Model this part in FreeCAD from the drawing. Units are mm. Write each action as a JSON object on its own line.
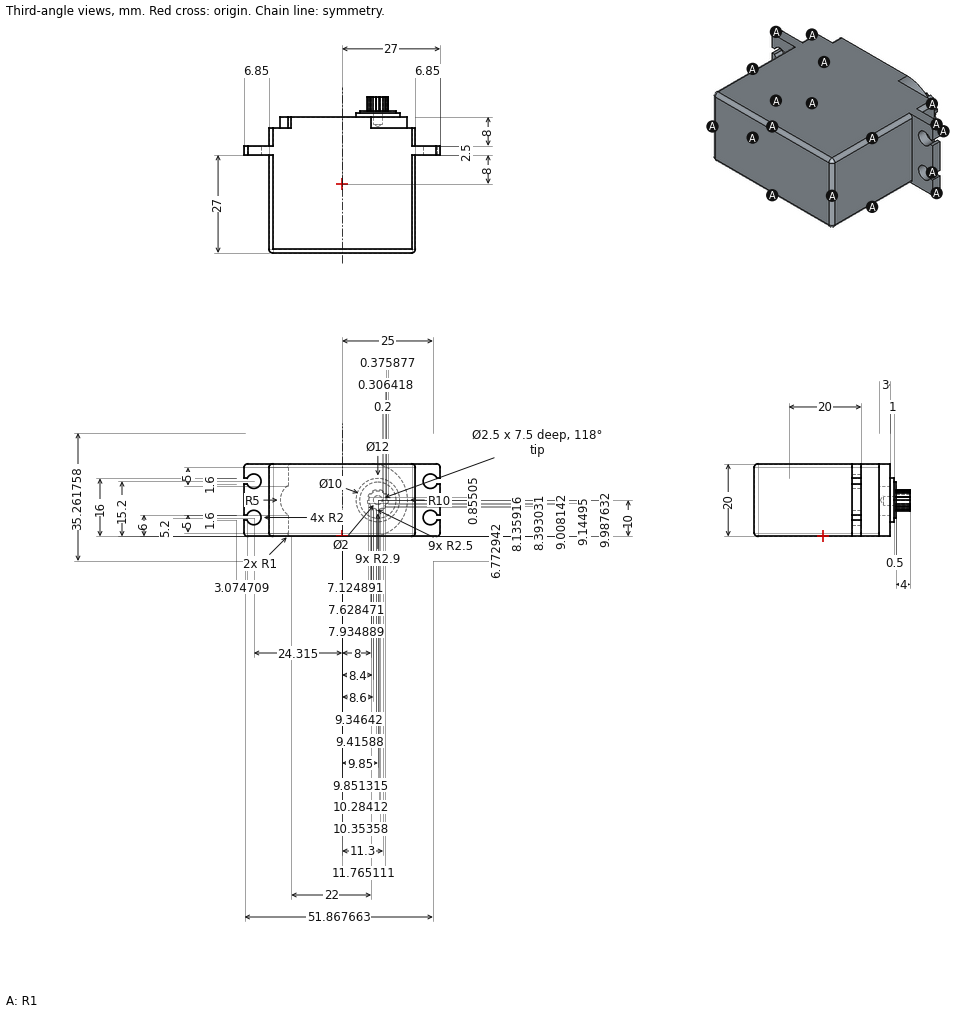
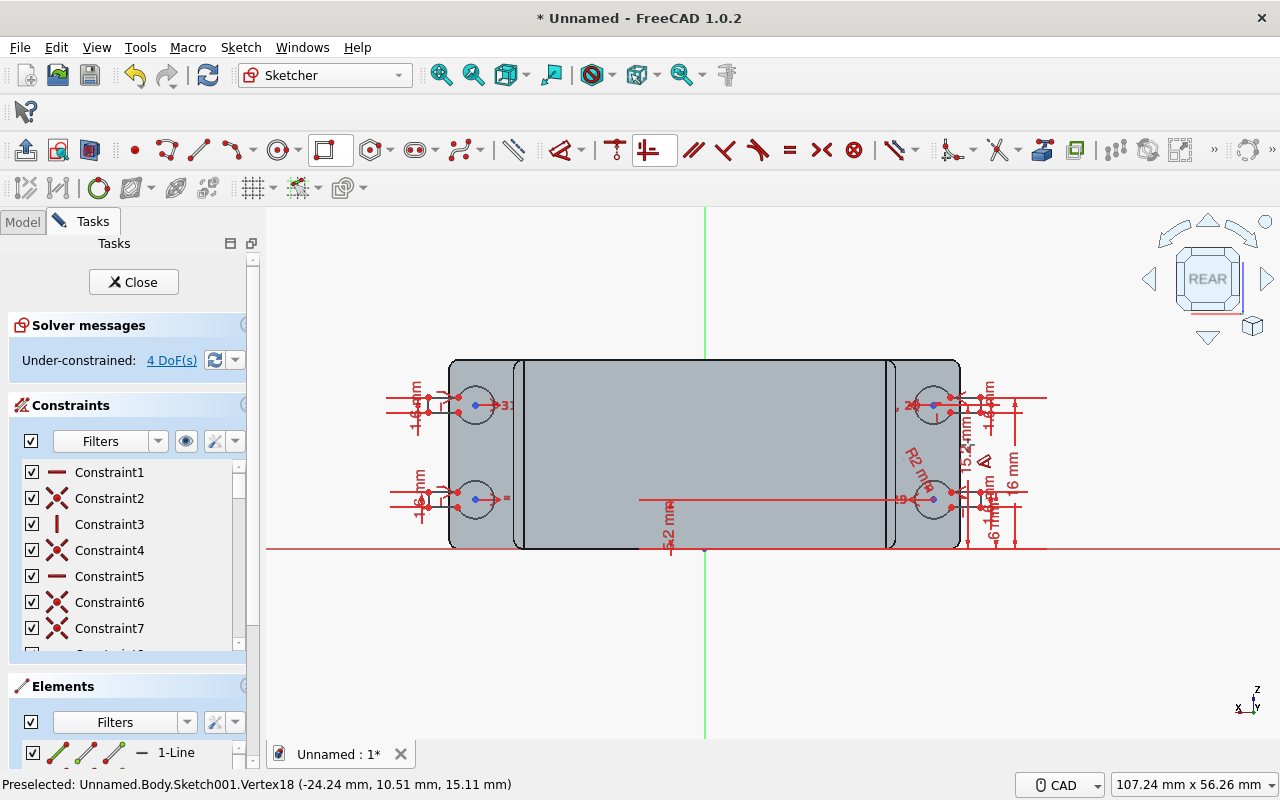
{"action": "left_click", "coordinate": [934, 500]}
{"action": "left_click", "coordinate": [819, 583]}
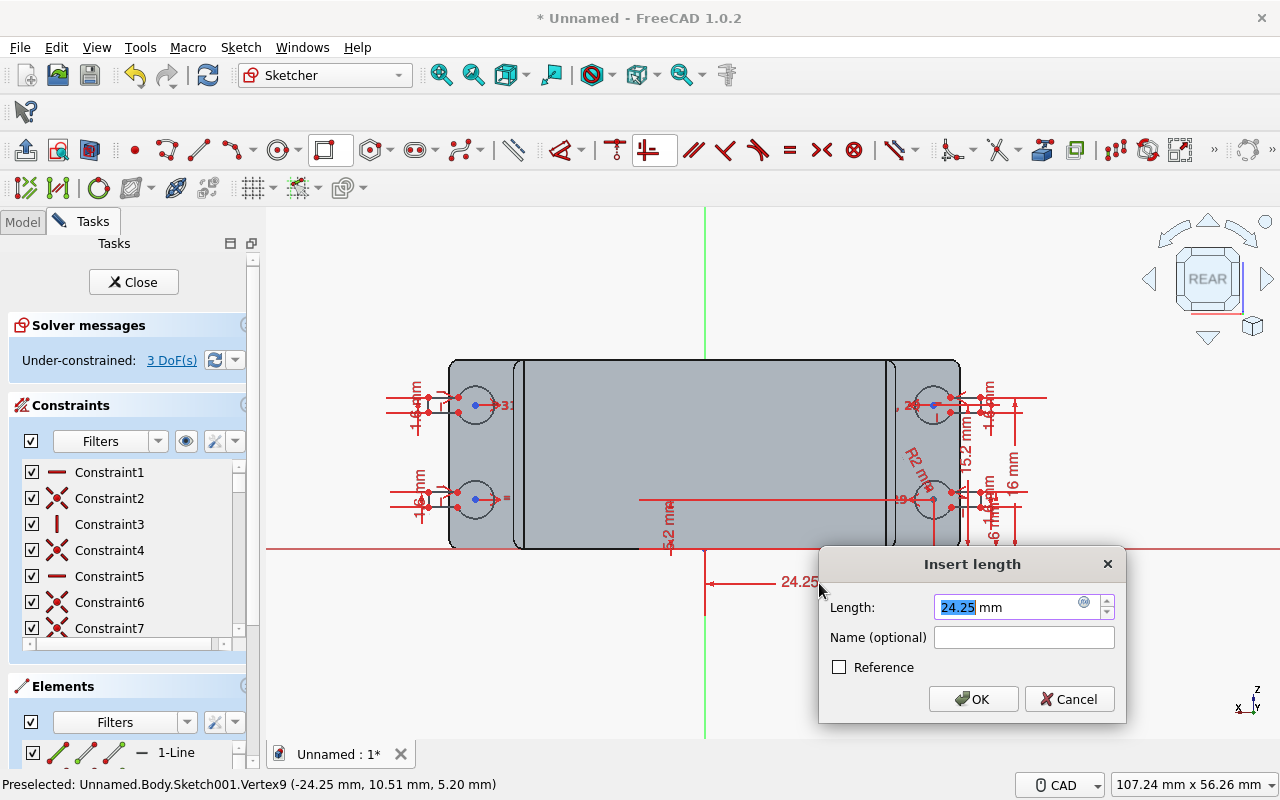
{"action": "type", "text": "24.315"}
{"action": "key", "text": "Return"}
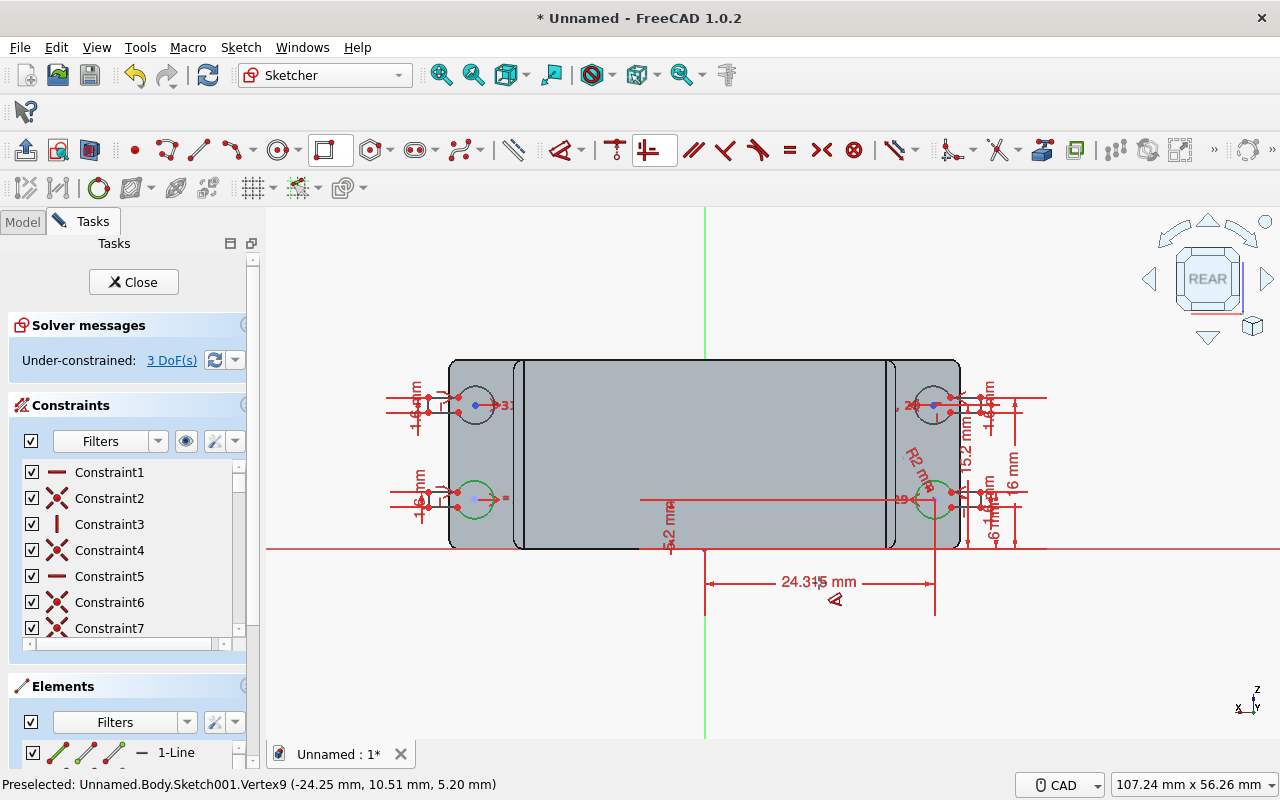
{"action": "left_click", "coordinate": [934, 405]}
{"action": "left_click", "coordinate": [739, 583]}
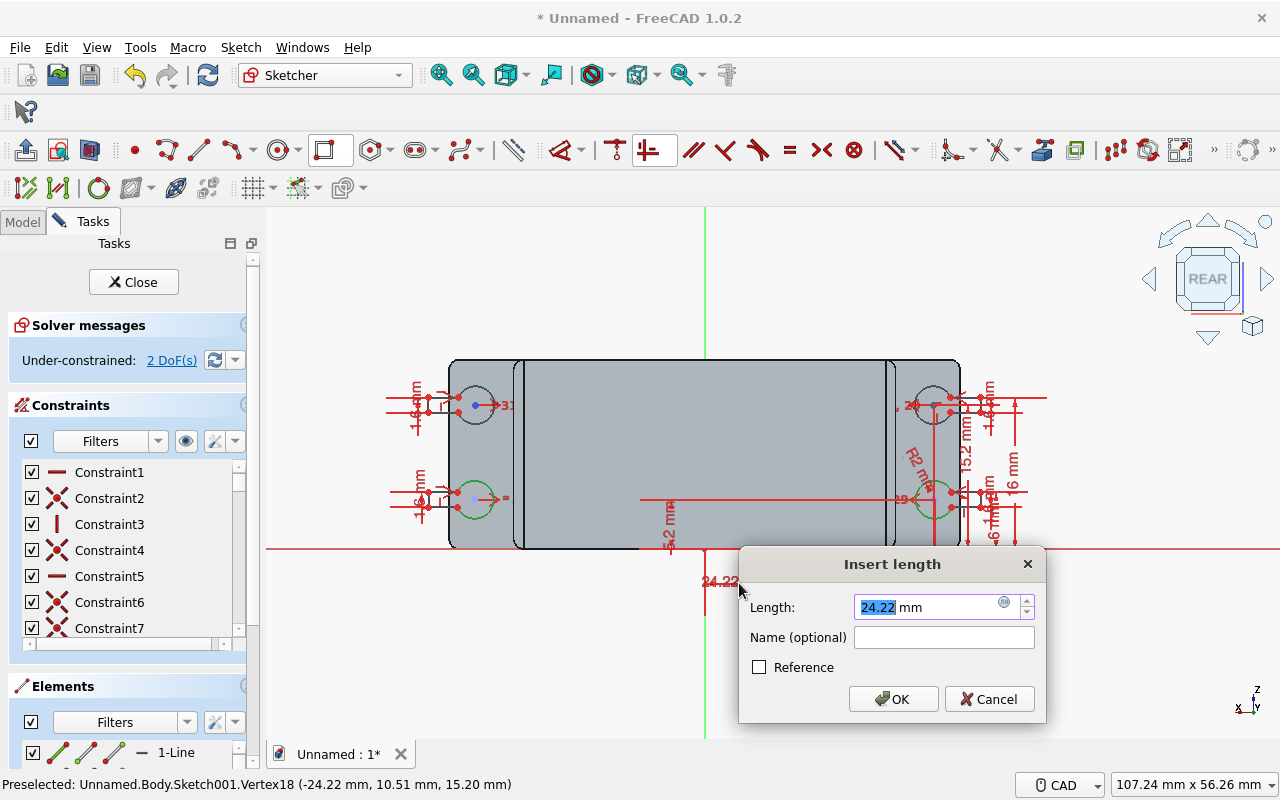
{"action": "type", "text": "24.315"}
{"action": "key", "text": "Return"}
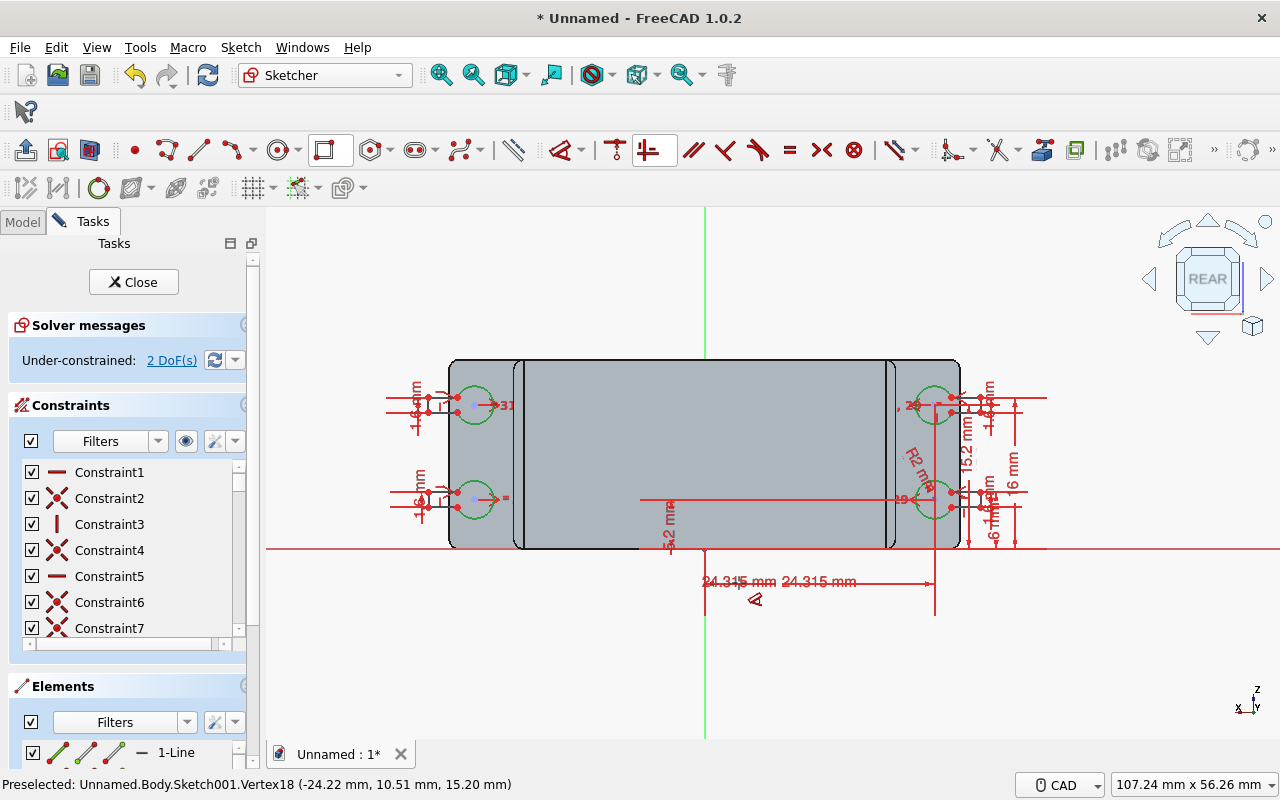
{"action": "scroll", "coordinate": [963, 507], "scroll_direction": "up", "scroll_amount": 2}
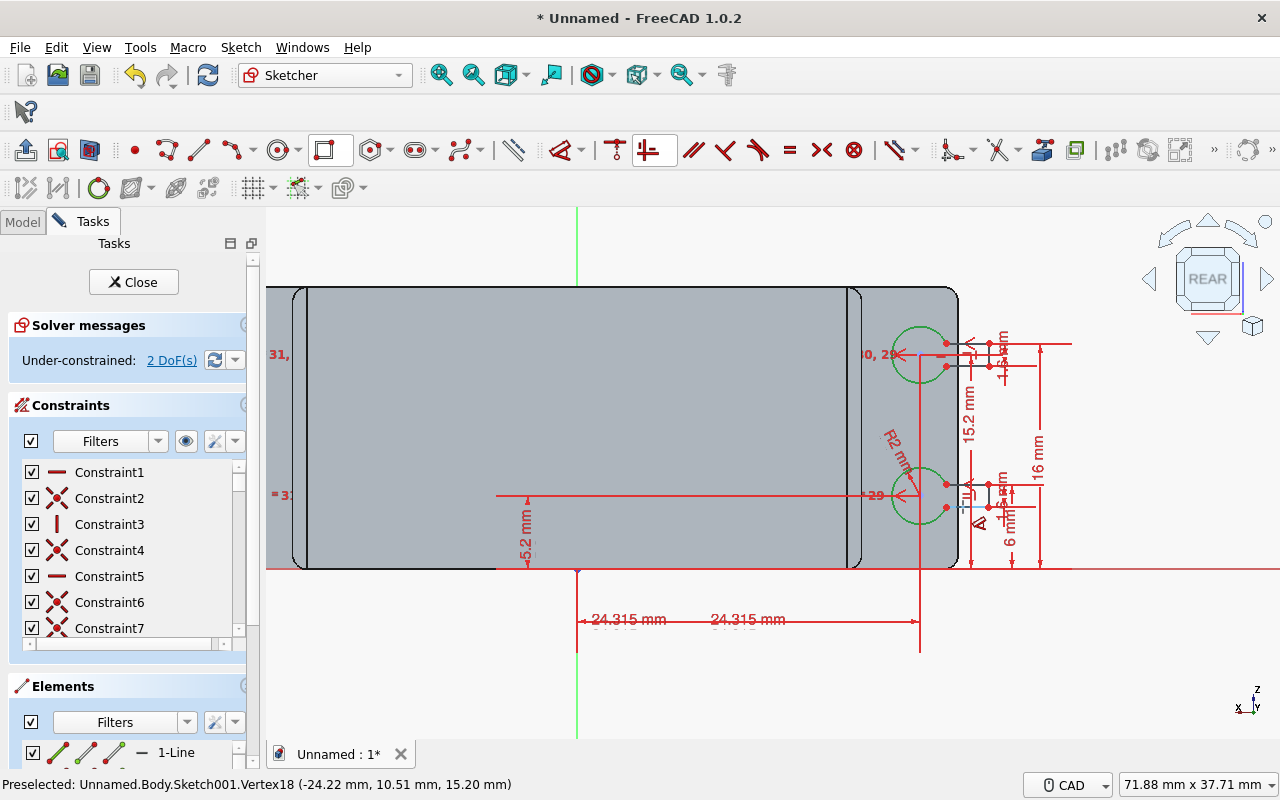
{"action": "left_click", "coordinate": [963, 507]}
{"action": "left_click", "coordinate": [968, 449]}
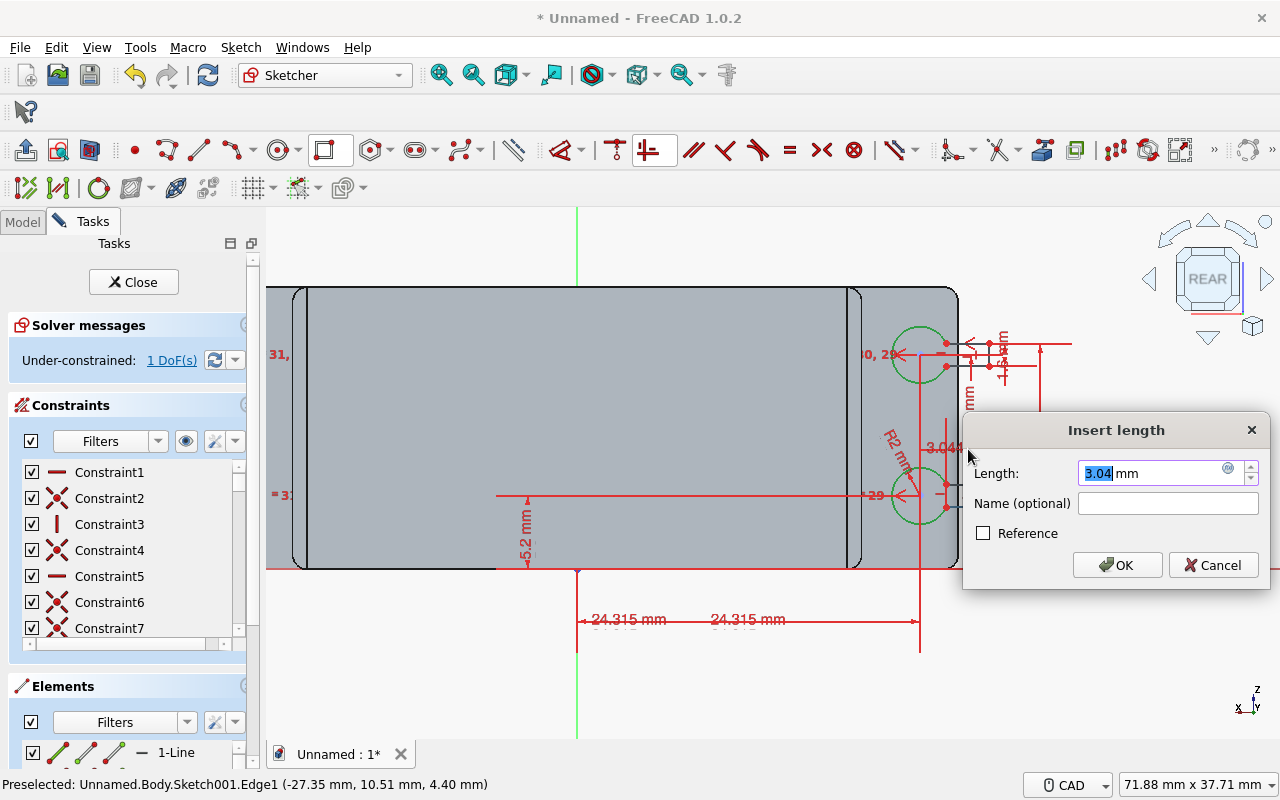
{"action": "type", "text": "3.074709"}
{"action": "key", "text": "Return"}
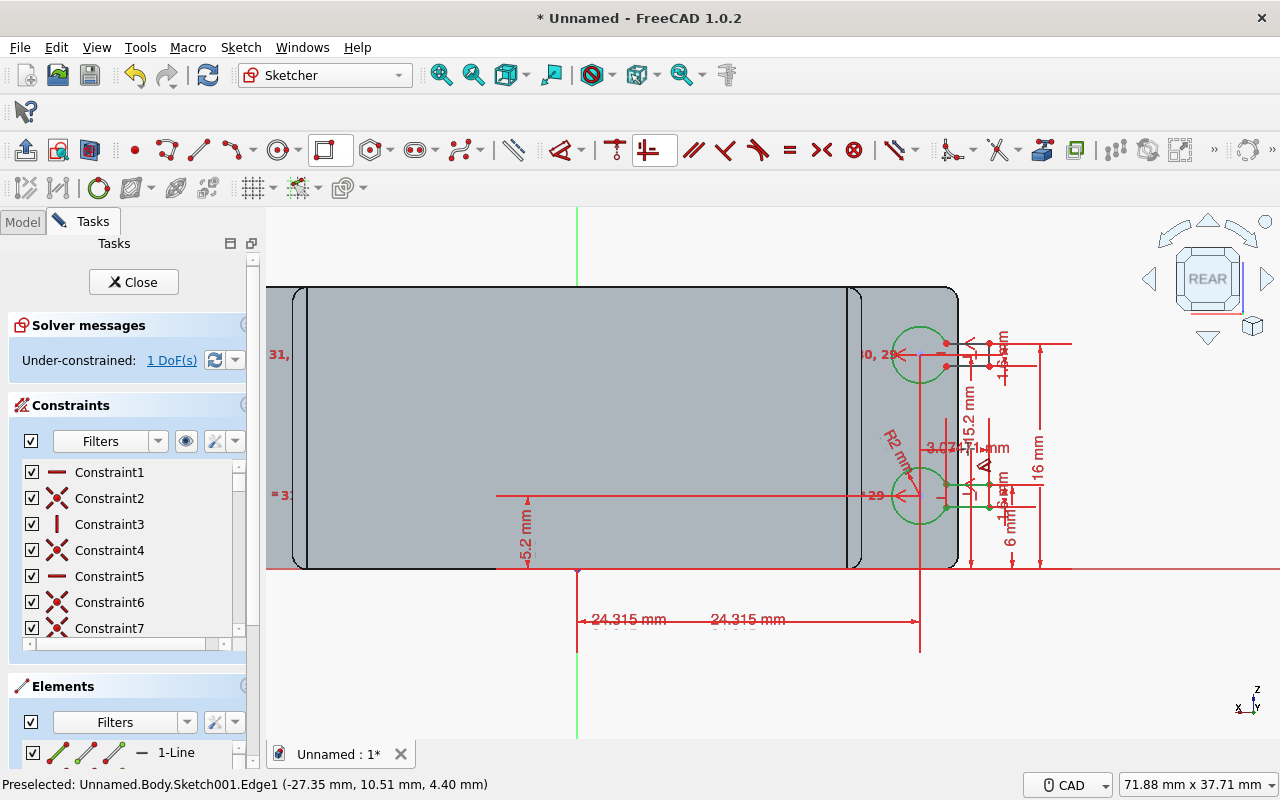
{"action": "left_click", "coordinate": [959, 366]}
{"action": "left_click", "coordinate": [968, 308]}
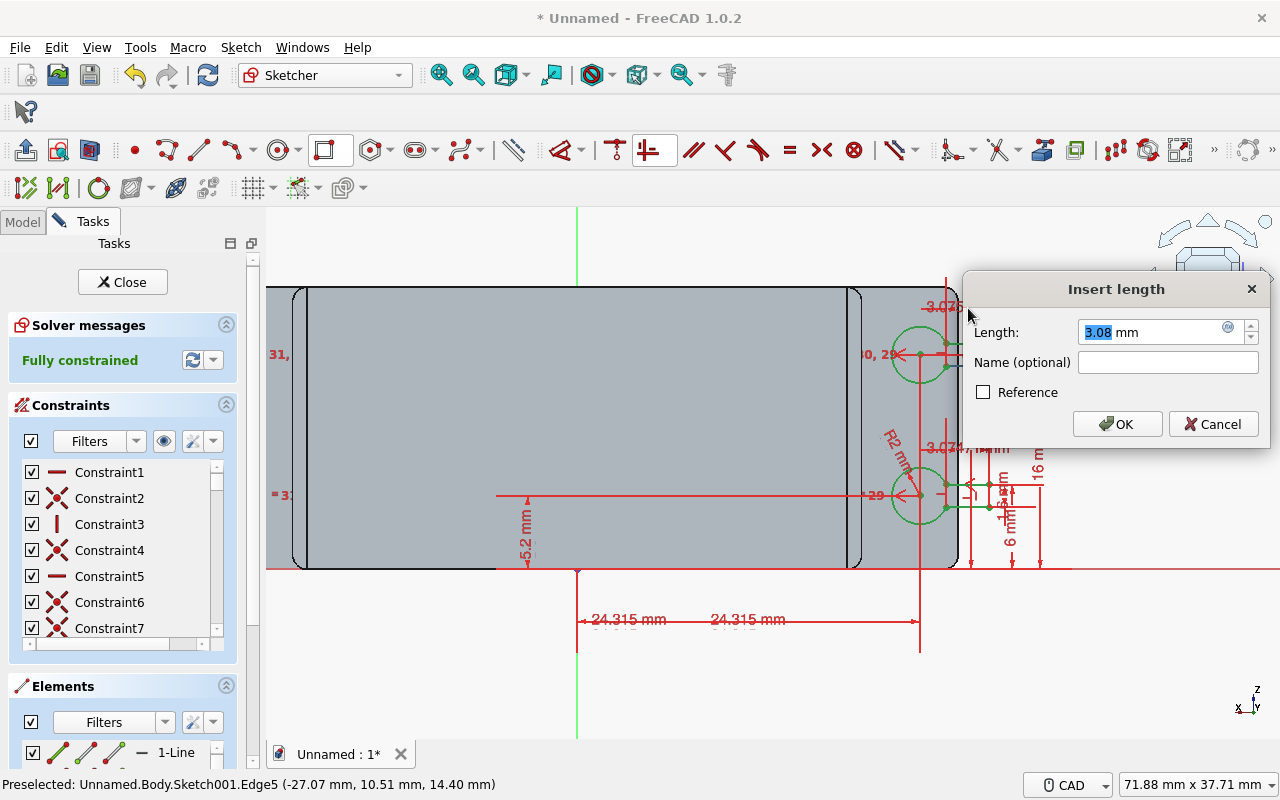
{"action": "type", "text": "3.074709"}
{"action": "key", "text": "Return"}
{"action": "key", "text": "Escape"}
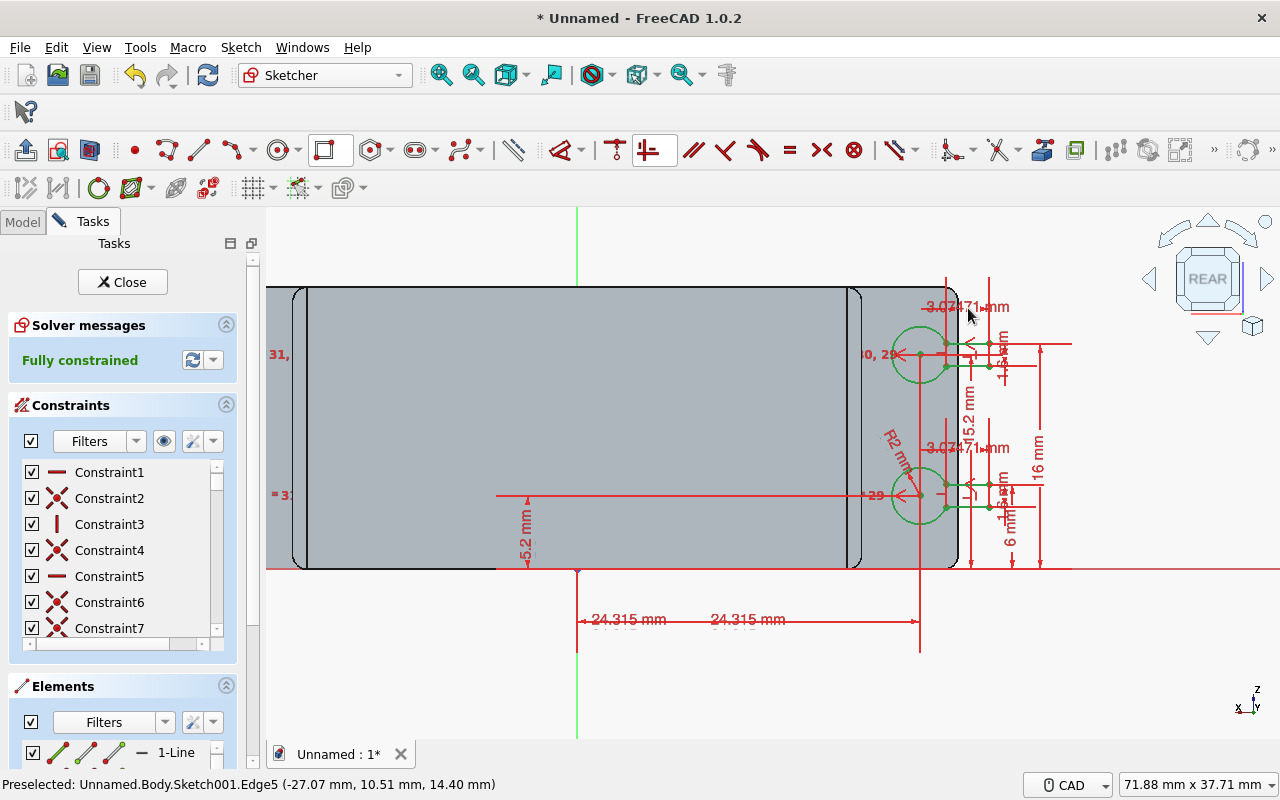
{"action": "left_click", "coordinate": [123, 282]}